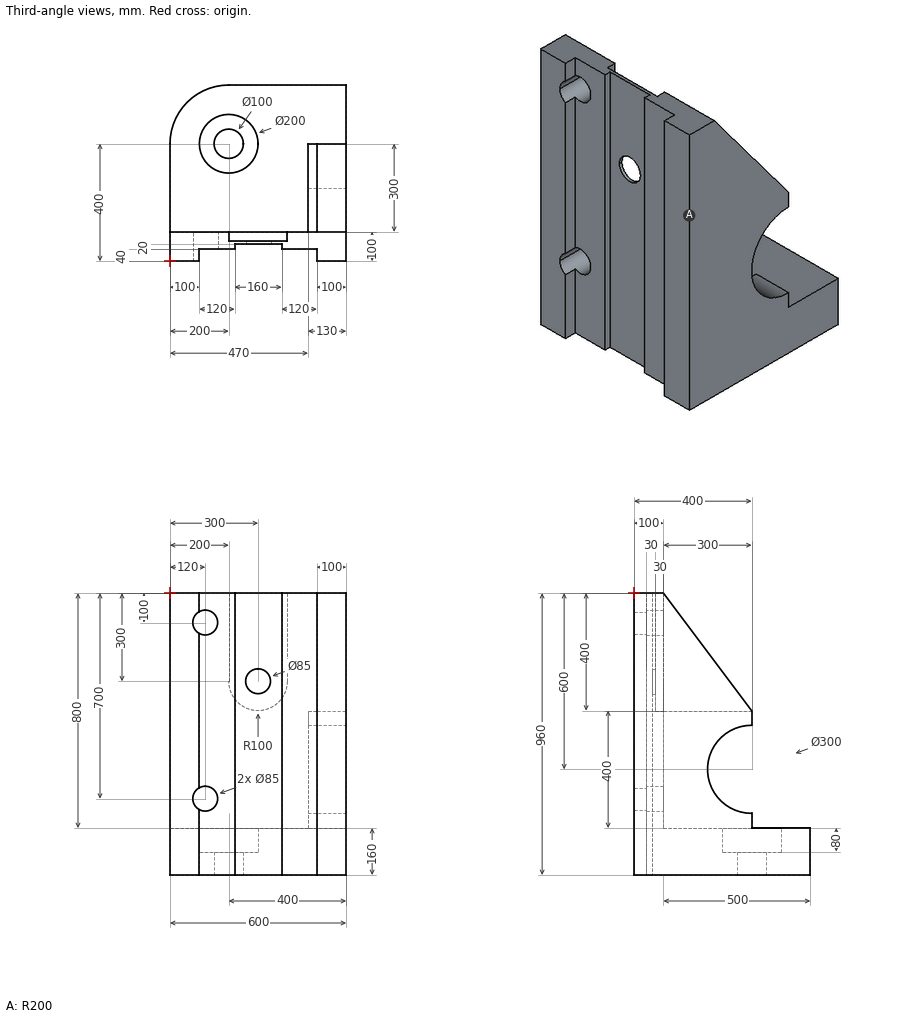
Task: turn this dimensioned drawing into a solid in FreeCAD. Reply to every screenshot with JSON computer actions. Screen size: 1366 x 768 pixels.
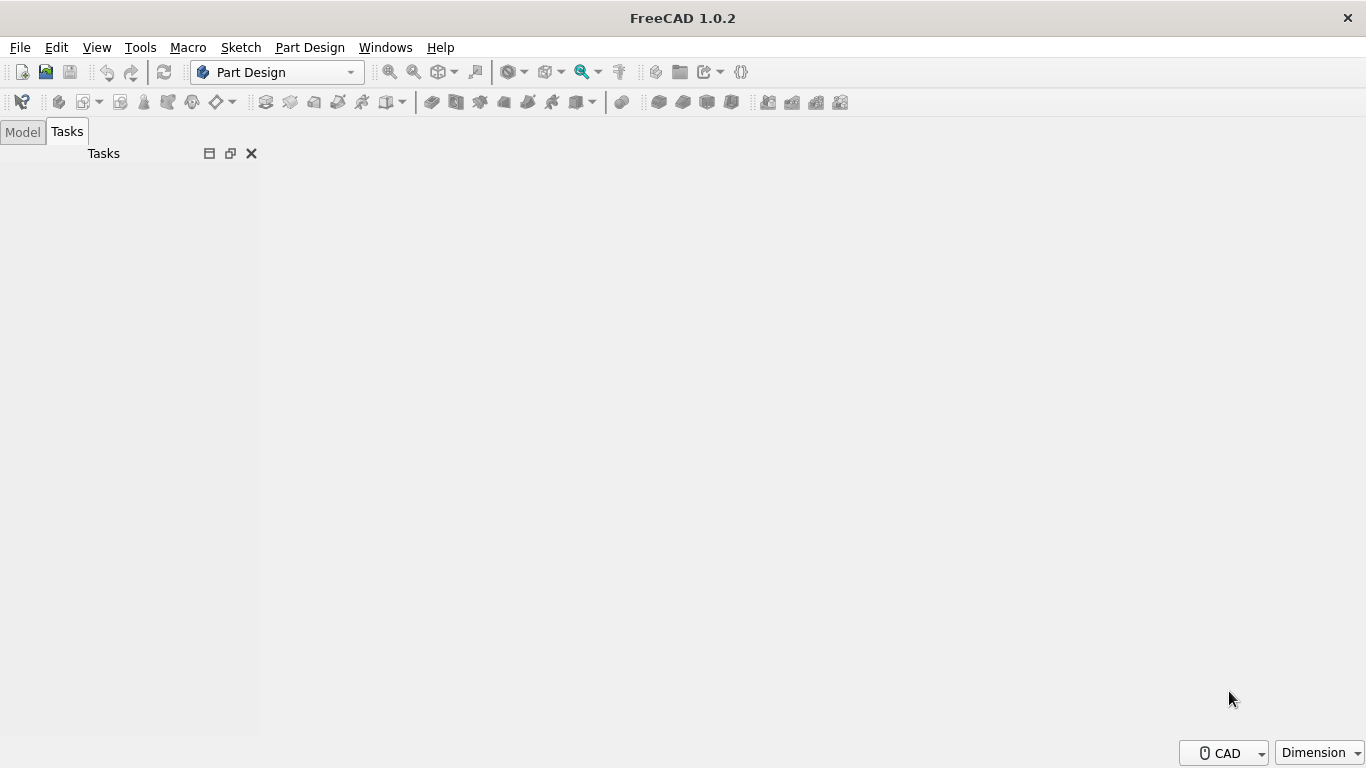
{"action": "left_click", "coordinate": [22, 72]}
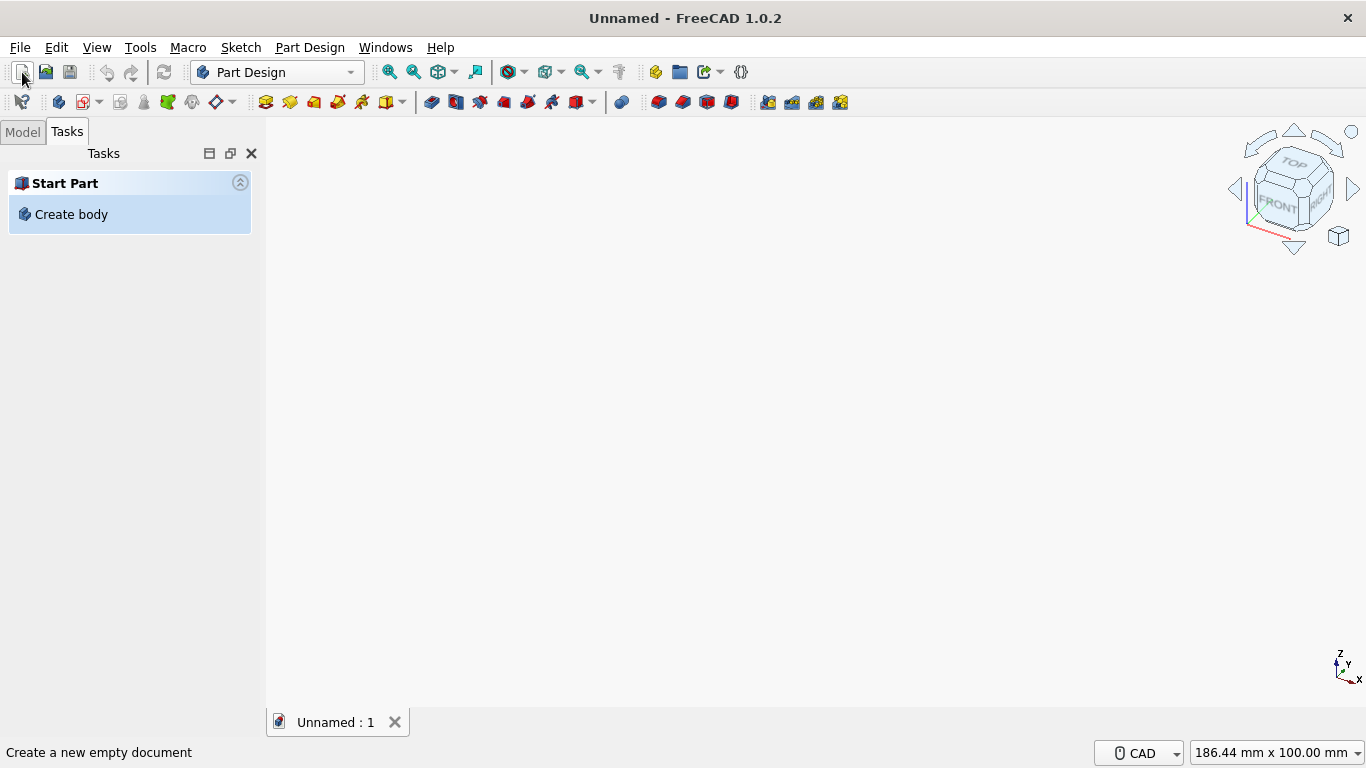
{"action": "left_click", "coordinate": [84, 102]}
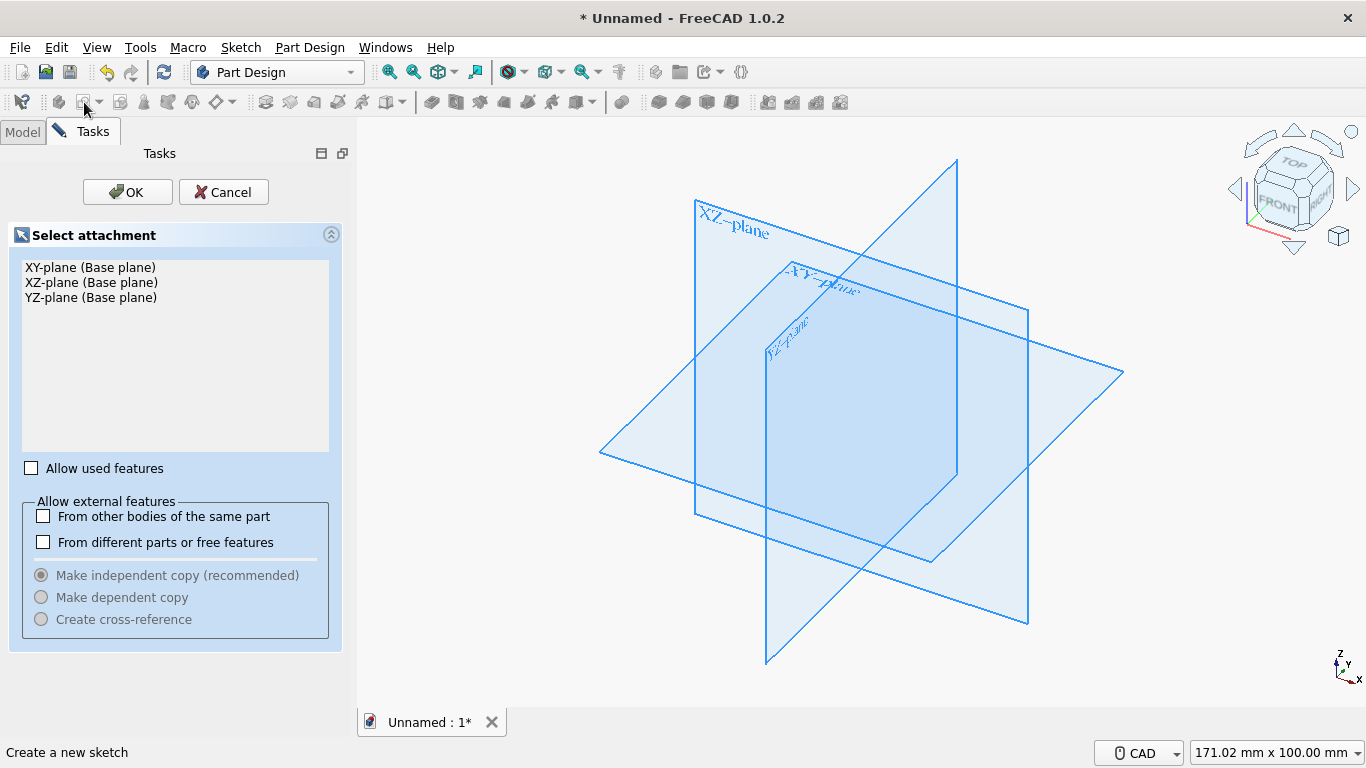
{"action": "left_click", "coordinate": [82, 268]}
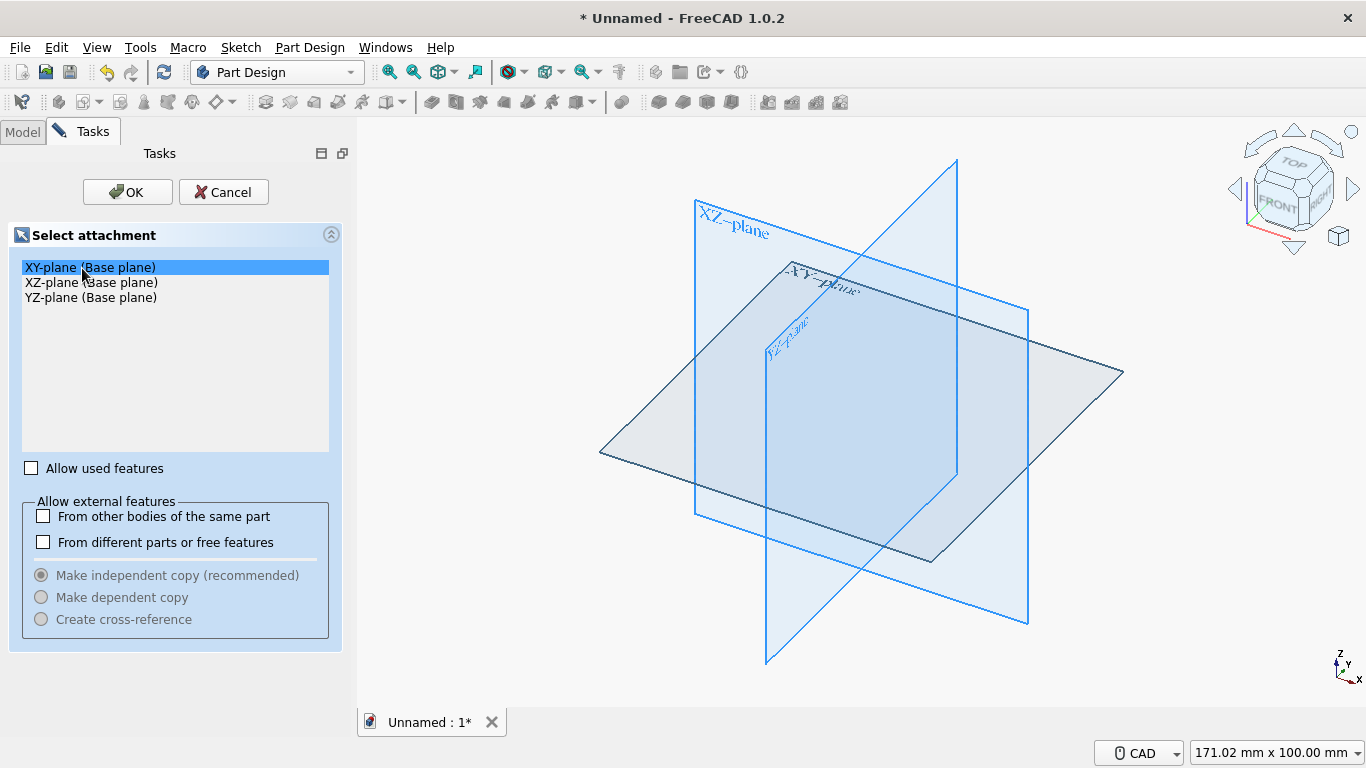
{"action": "left_click", "coordinate": [128, 192]}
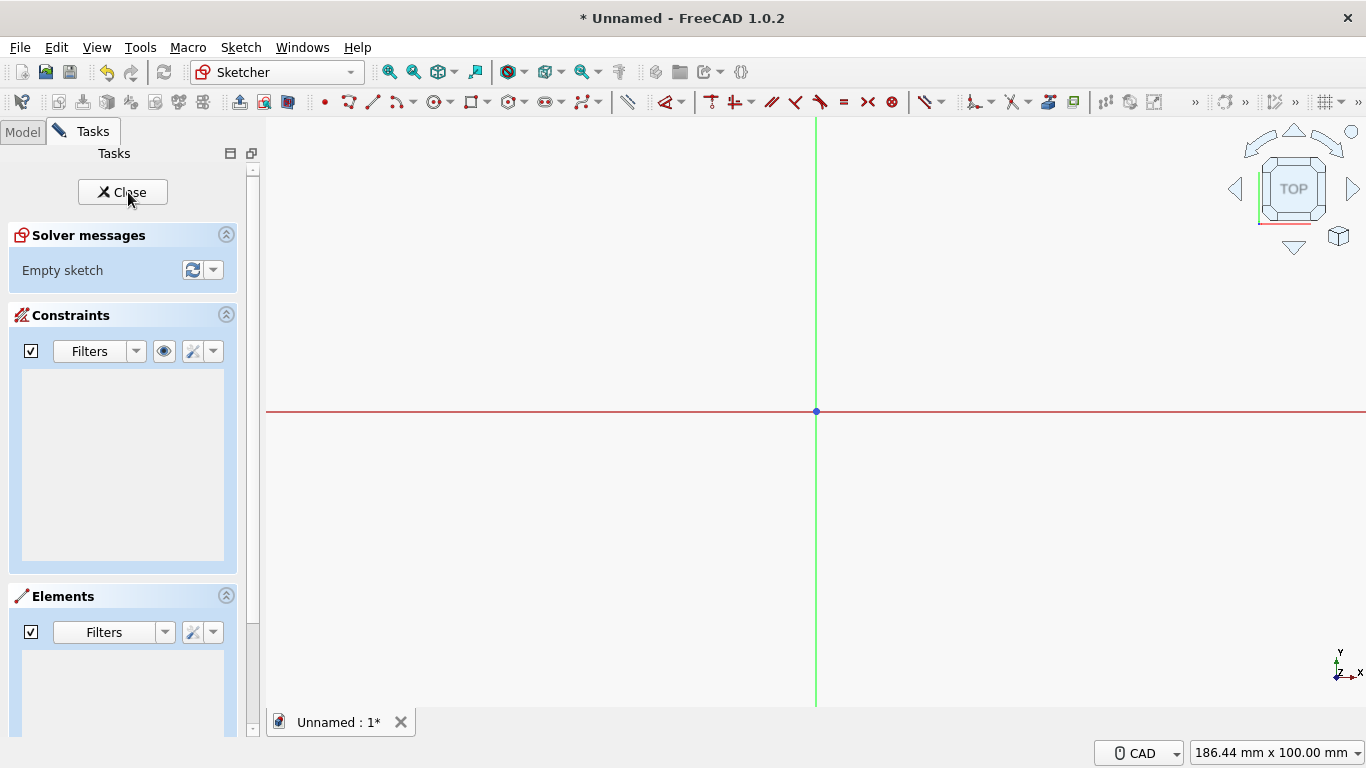
{"action": "scroll", "coordinate": [383, 470], "scroll_direction": "down", "scroll_amount": 9}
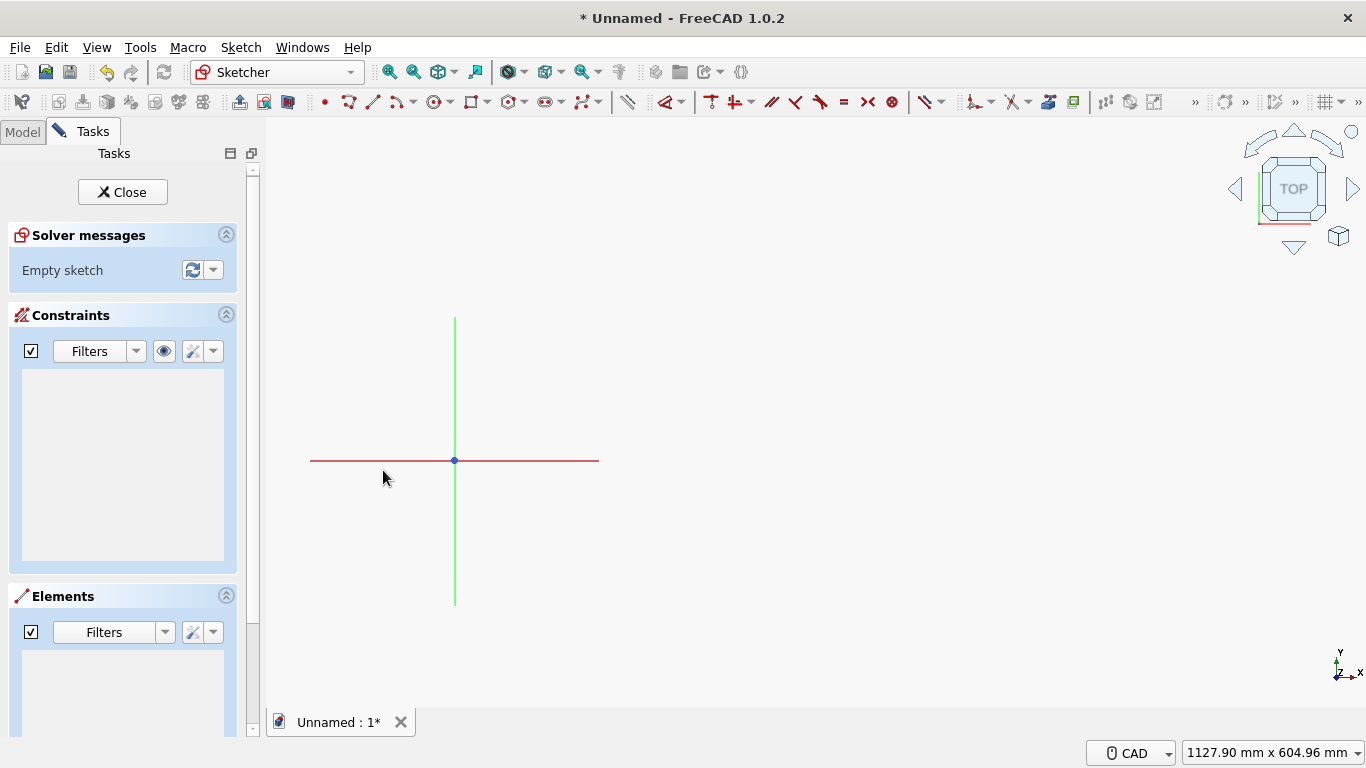
{"action": "left_click", "coordinate": [350, 102]}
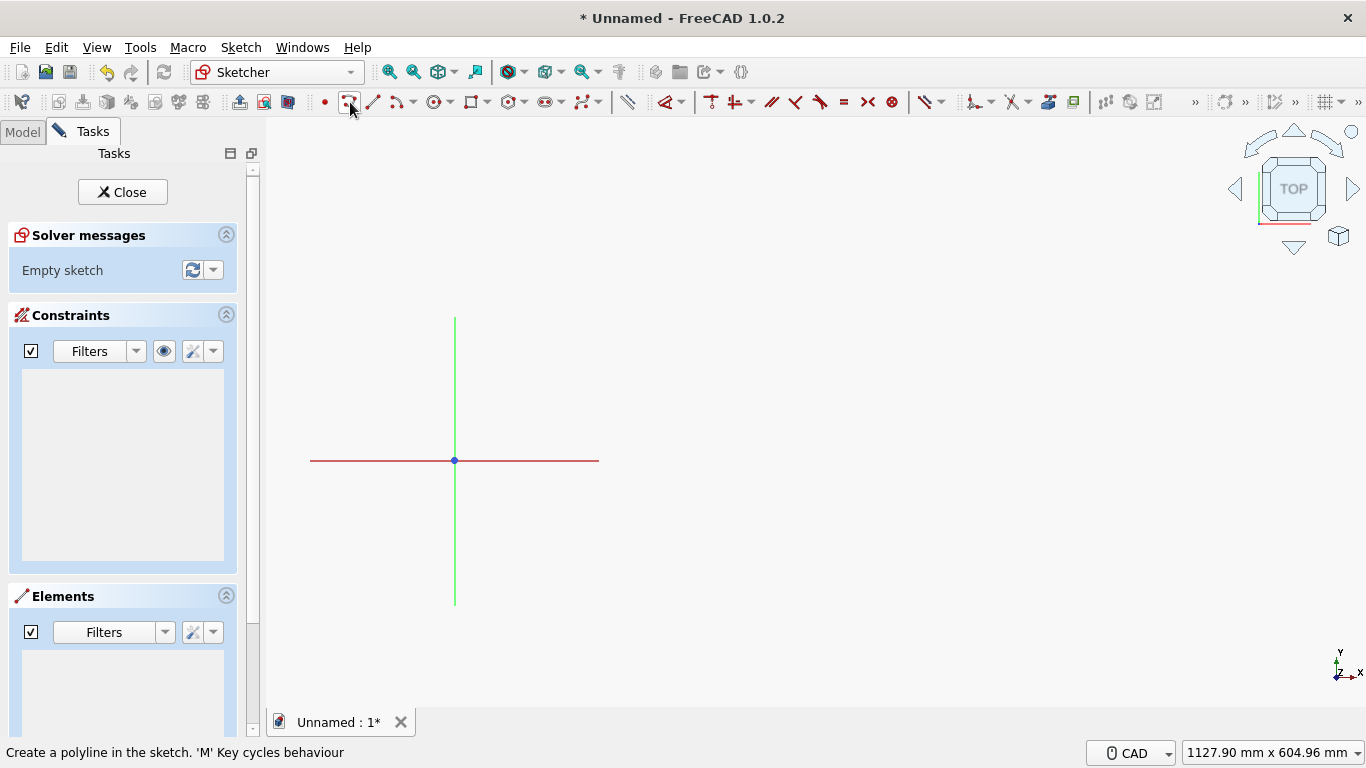
{"action": "left_click", "coordinate": [455, 461]}
{"action": "left_click", "coordinate": [552, 452]}
{"action": "left_click", "coordinate": [552, 422]}
{"action": "left_click", "coordinate": [669, 422]}
{"action": "left_click", "coordinate": [669, 402]}
{"action": "left_click", "coordinate": [825, 402]}
{"action": "left_click", "coordinate": [825, 422]}
{"action": "left_click", "coordinate": [942, 422]}
{"action": "left_click", "coordinate": [942, 461]}
{"action": "left_click", "coordinate": [1040, 452]}
{"action": "left_click", "coordinate": [1040, 363]}
{"action": "left_click", "coordinate": [464, 363]}
{"action": "left_click", "coordinate": [455, 461]}
{"action": "key", "text": "Escape"}
{"action": "key", "text": "Escape"}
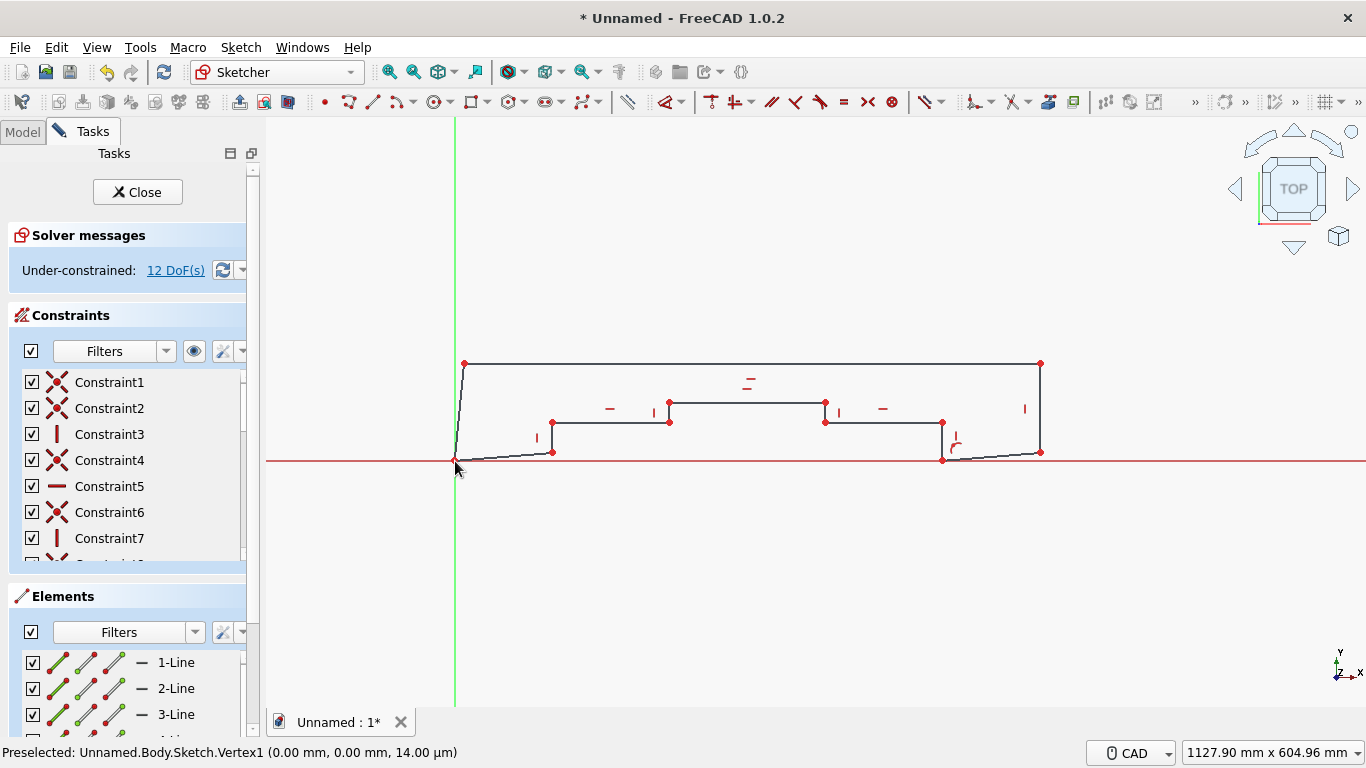
{"action": "left_click", "coordinate": [484, 459]}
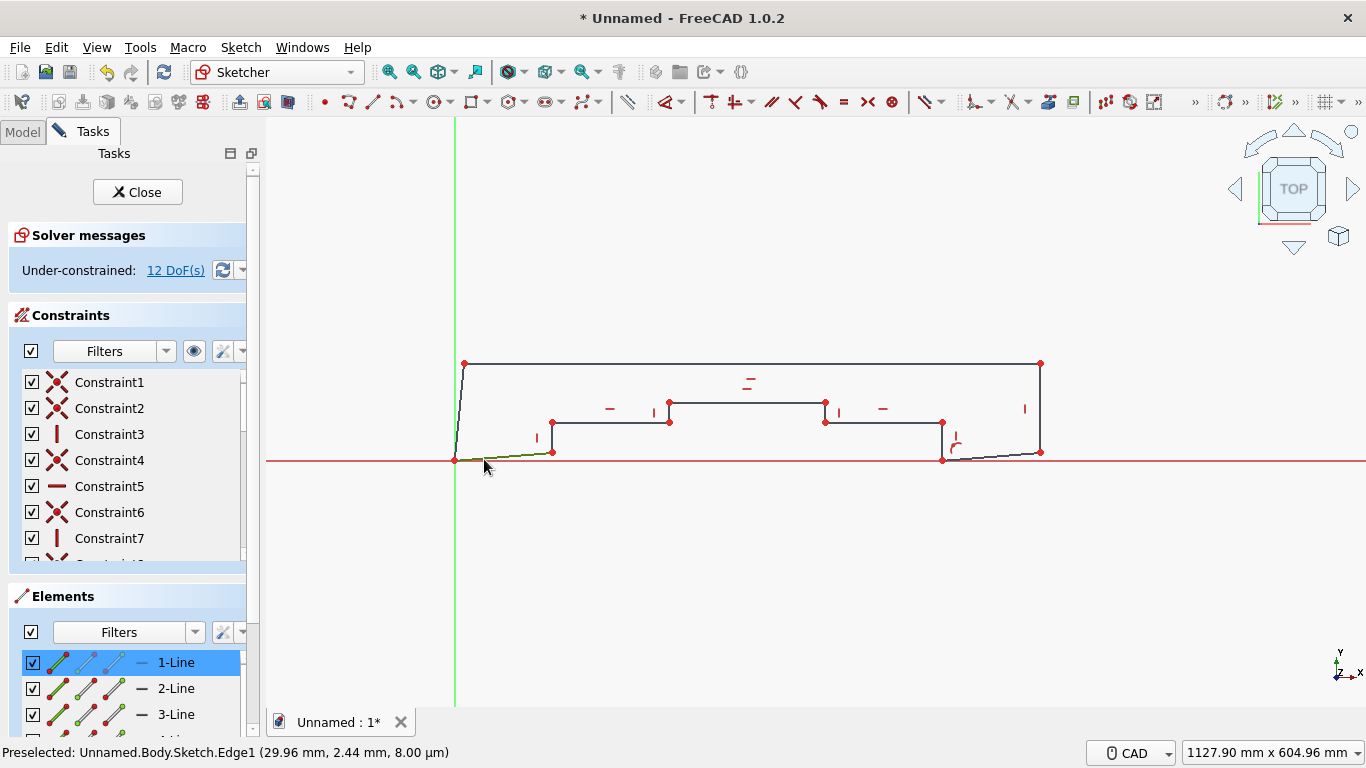
{"action": "left_click", "coordinate": [754, 102]}